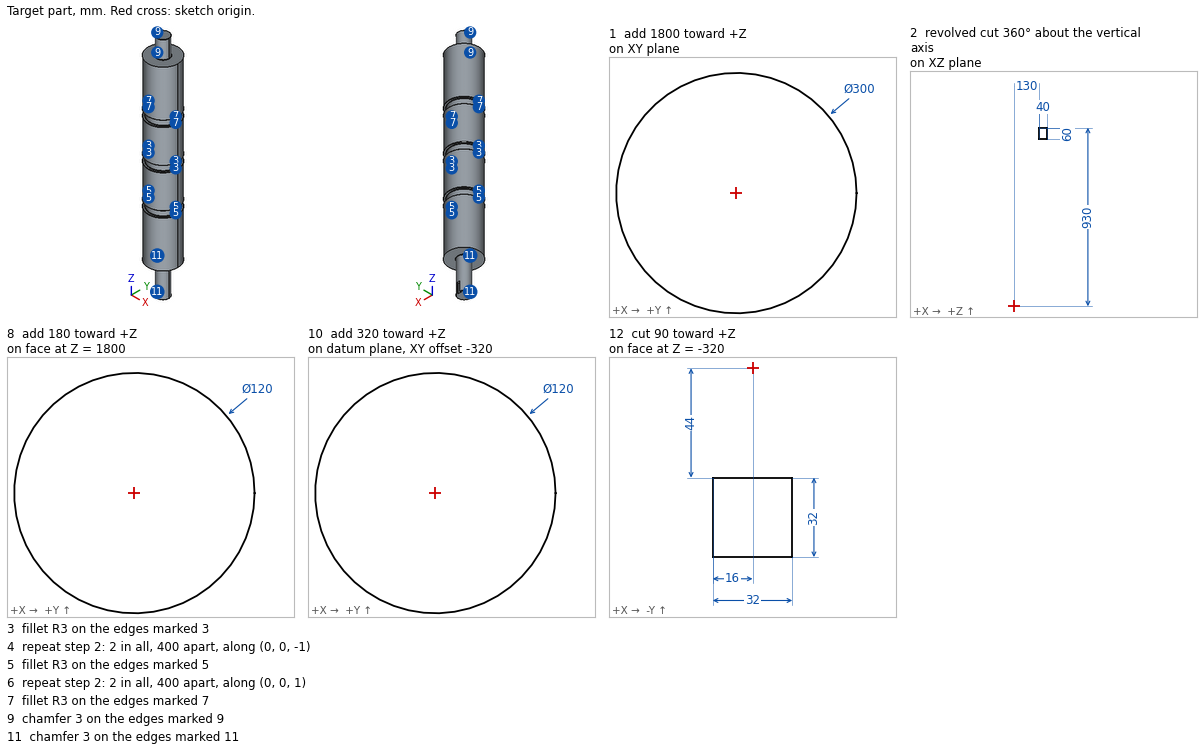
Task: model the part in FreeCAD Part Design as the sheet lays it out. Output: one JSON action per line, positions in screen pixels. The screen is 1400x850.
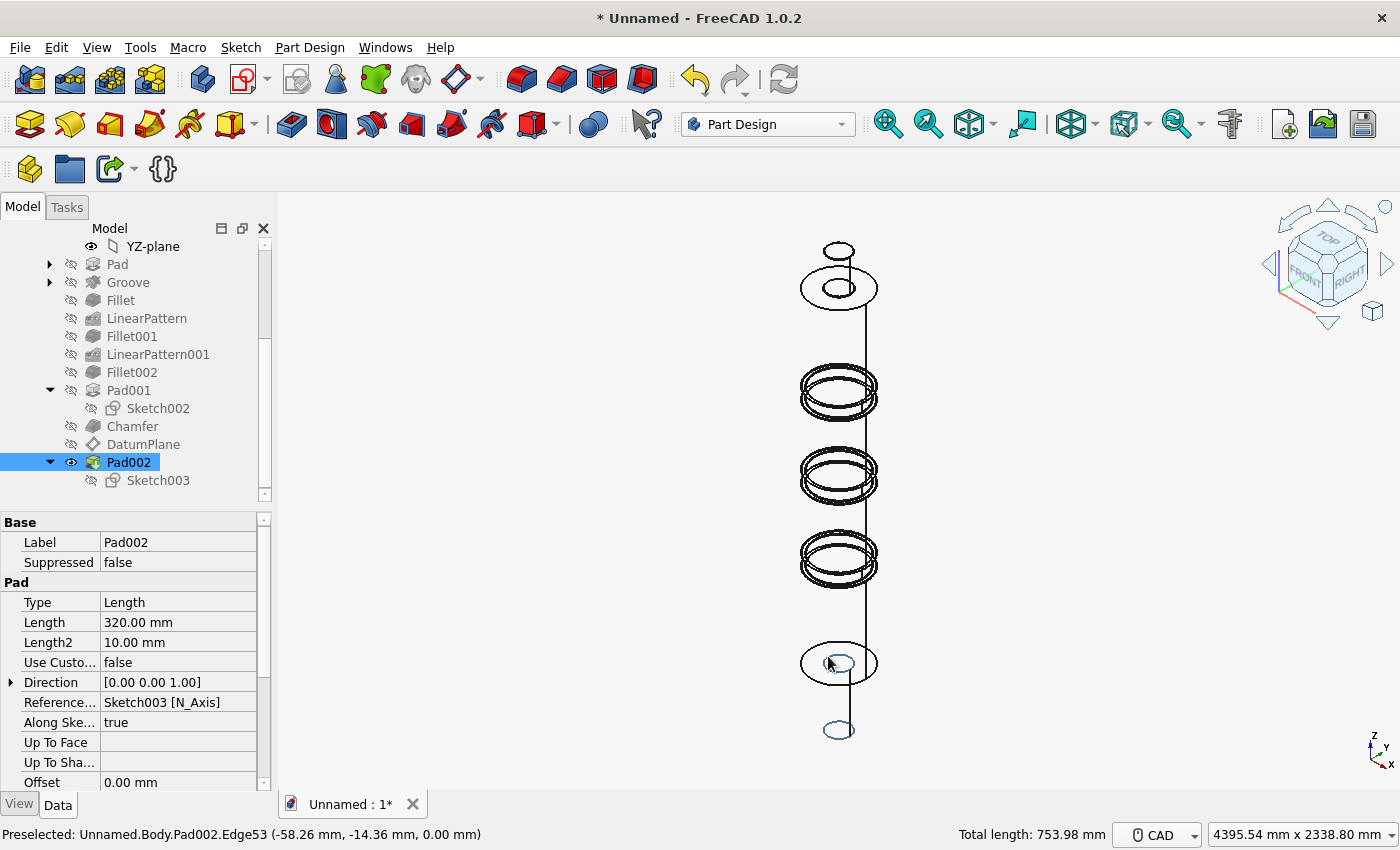
{"action": "key", "text": "v 1"}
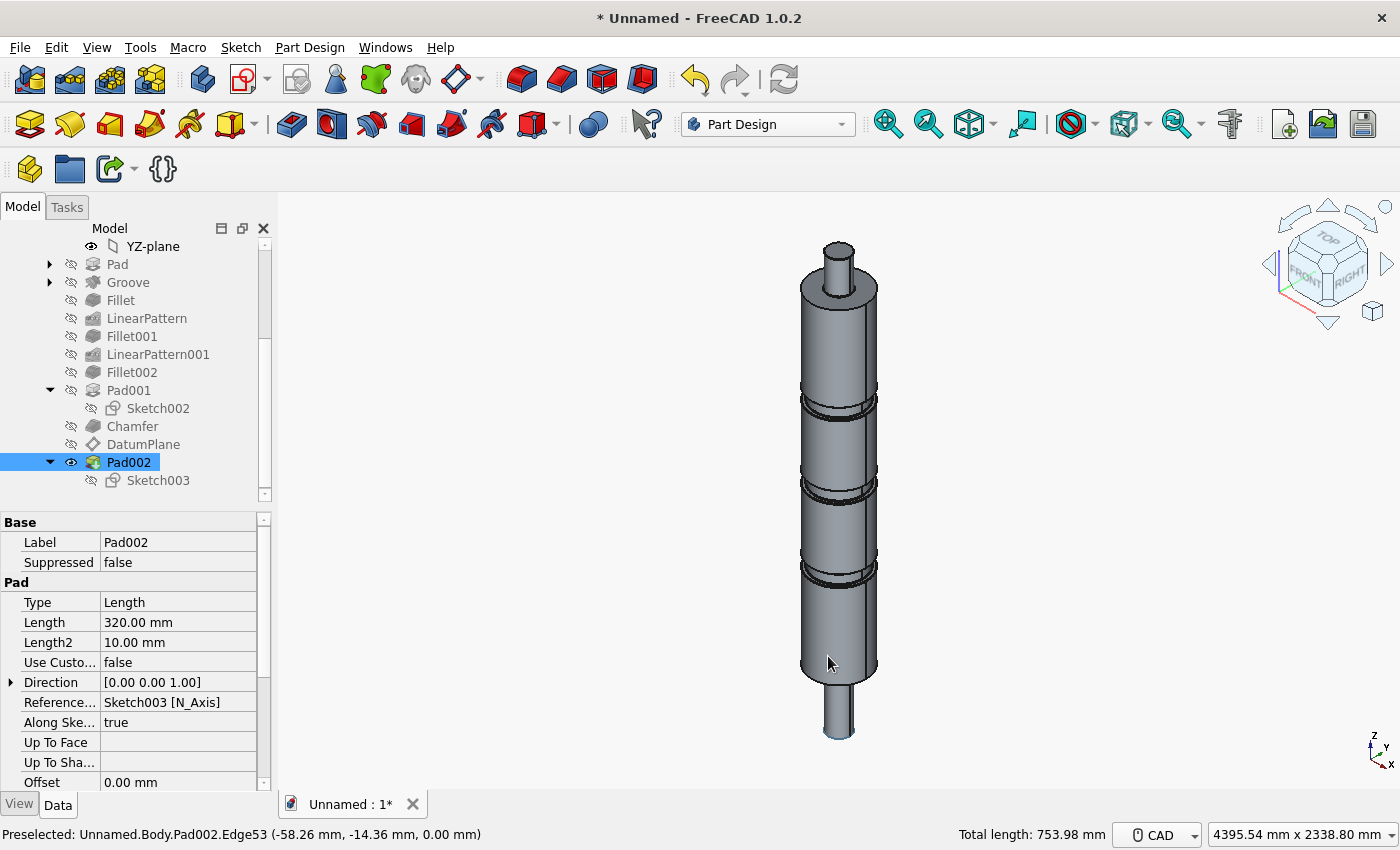
{"action": "left_click", "coordinate": [562, 80]}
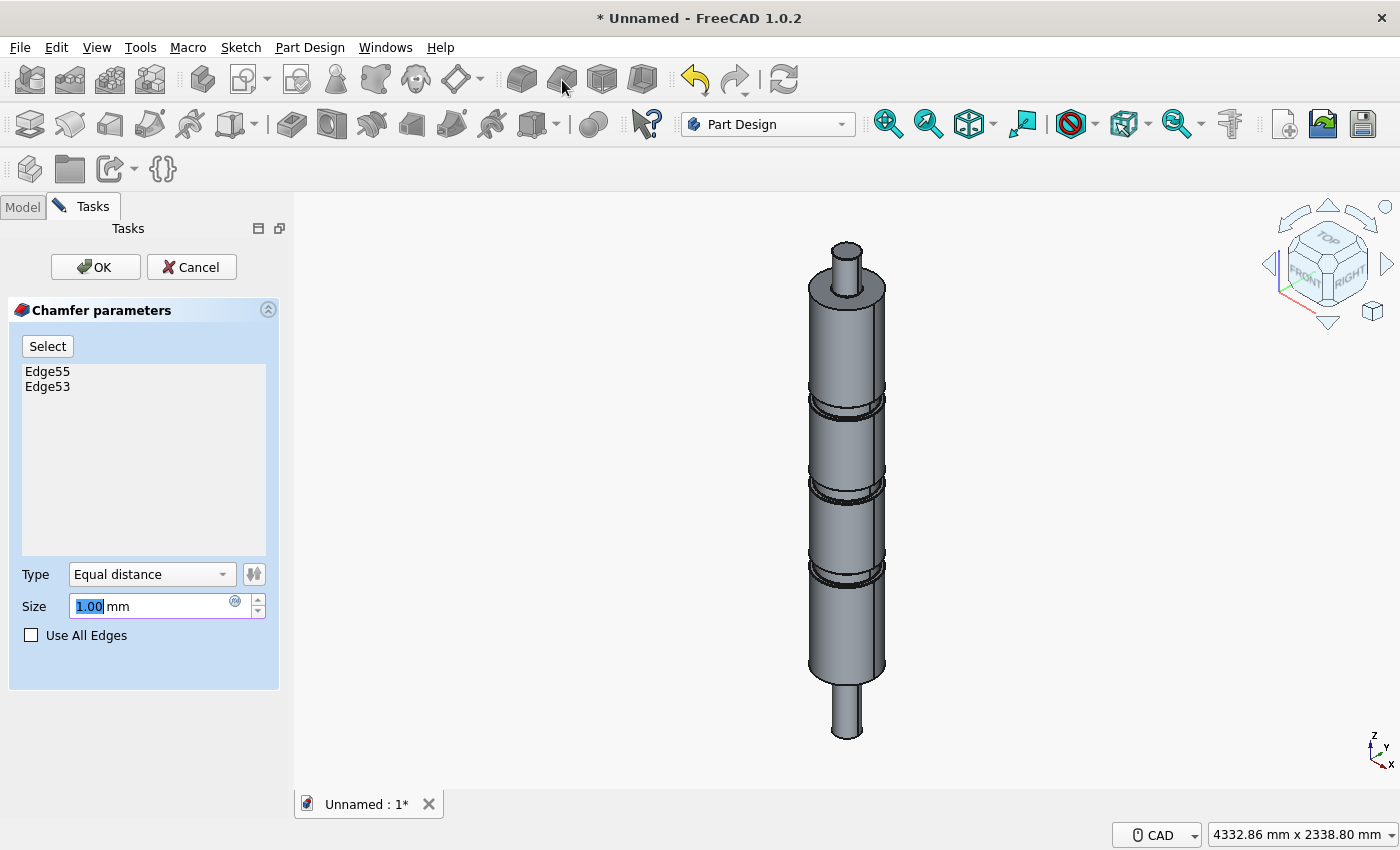
{"action": "type", "text": "3"}
{"action": "key", "text": "Tab"}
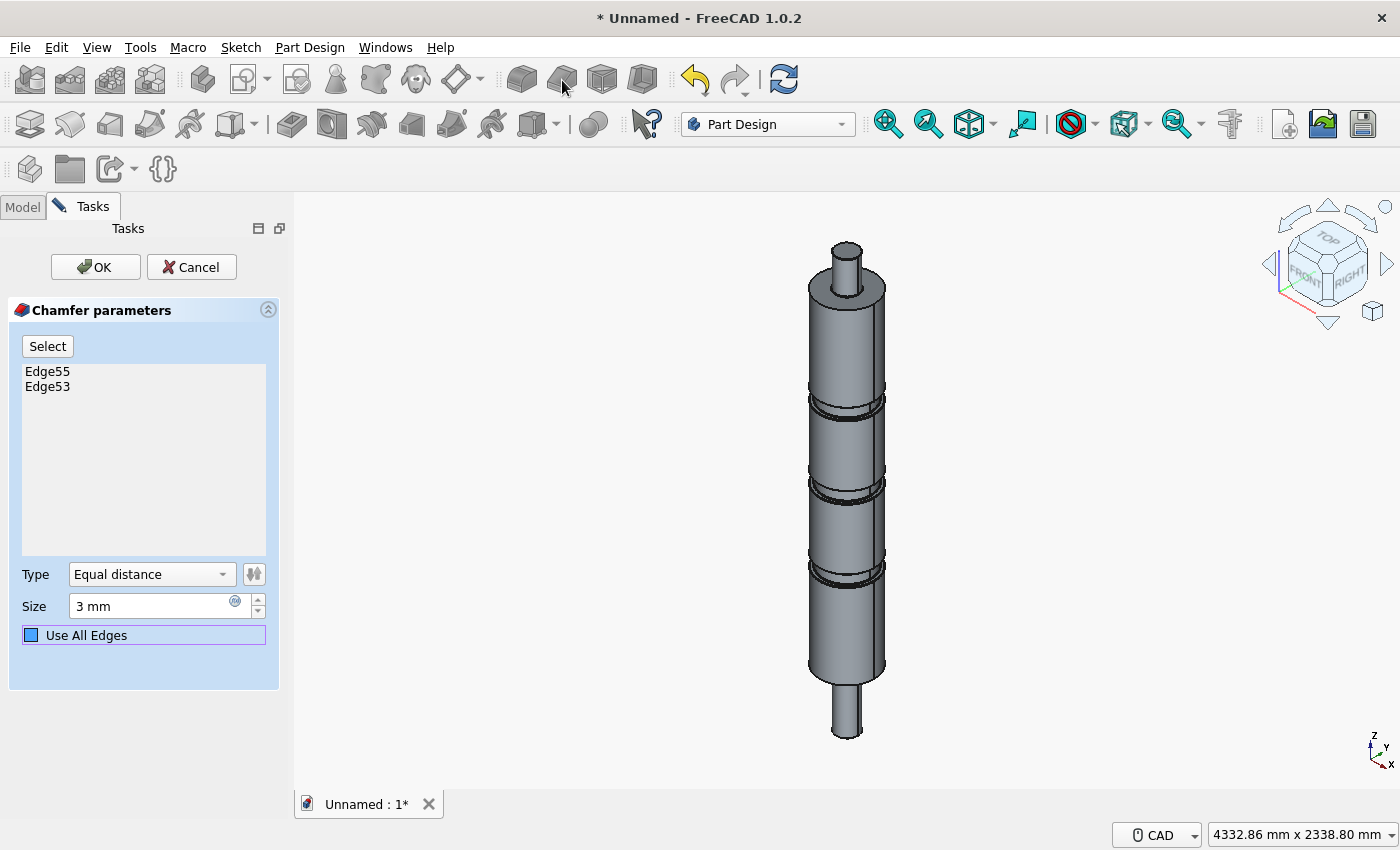
{"action": "left_click", "coordinate": [96, 267]}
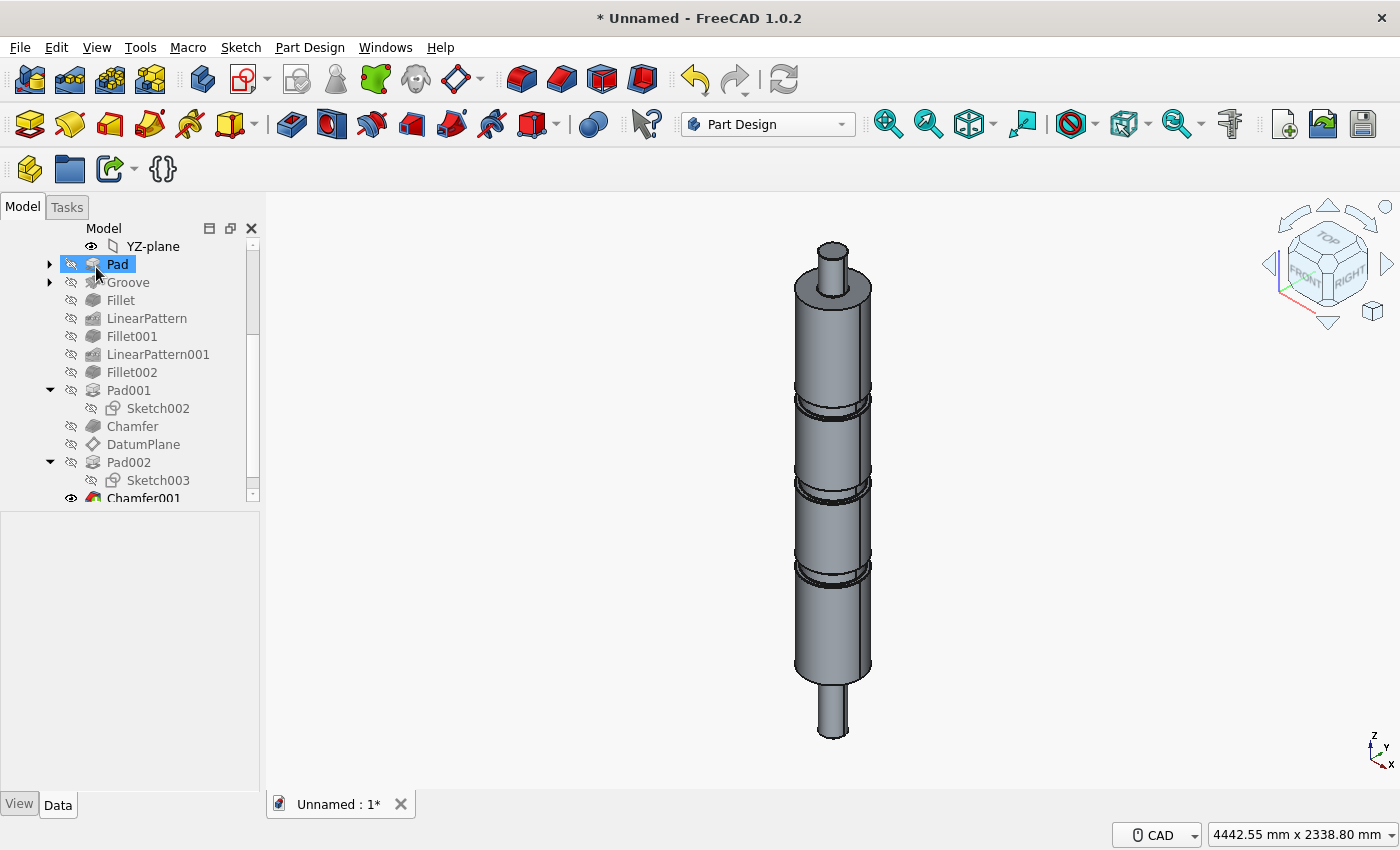
{"action": "key", "text": "5"}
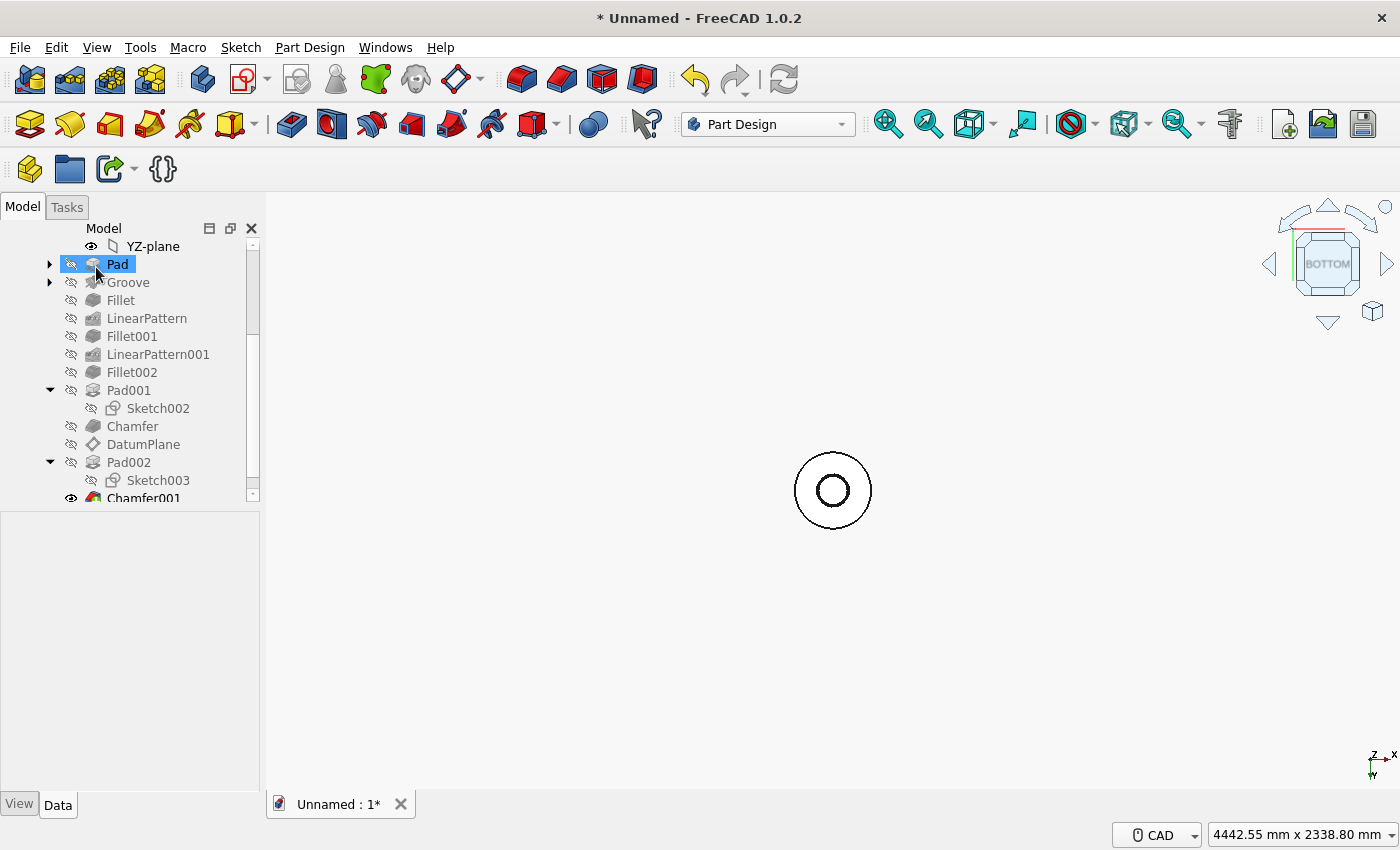
{"action": "left_click", "coordinate": [890, 124]}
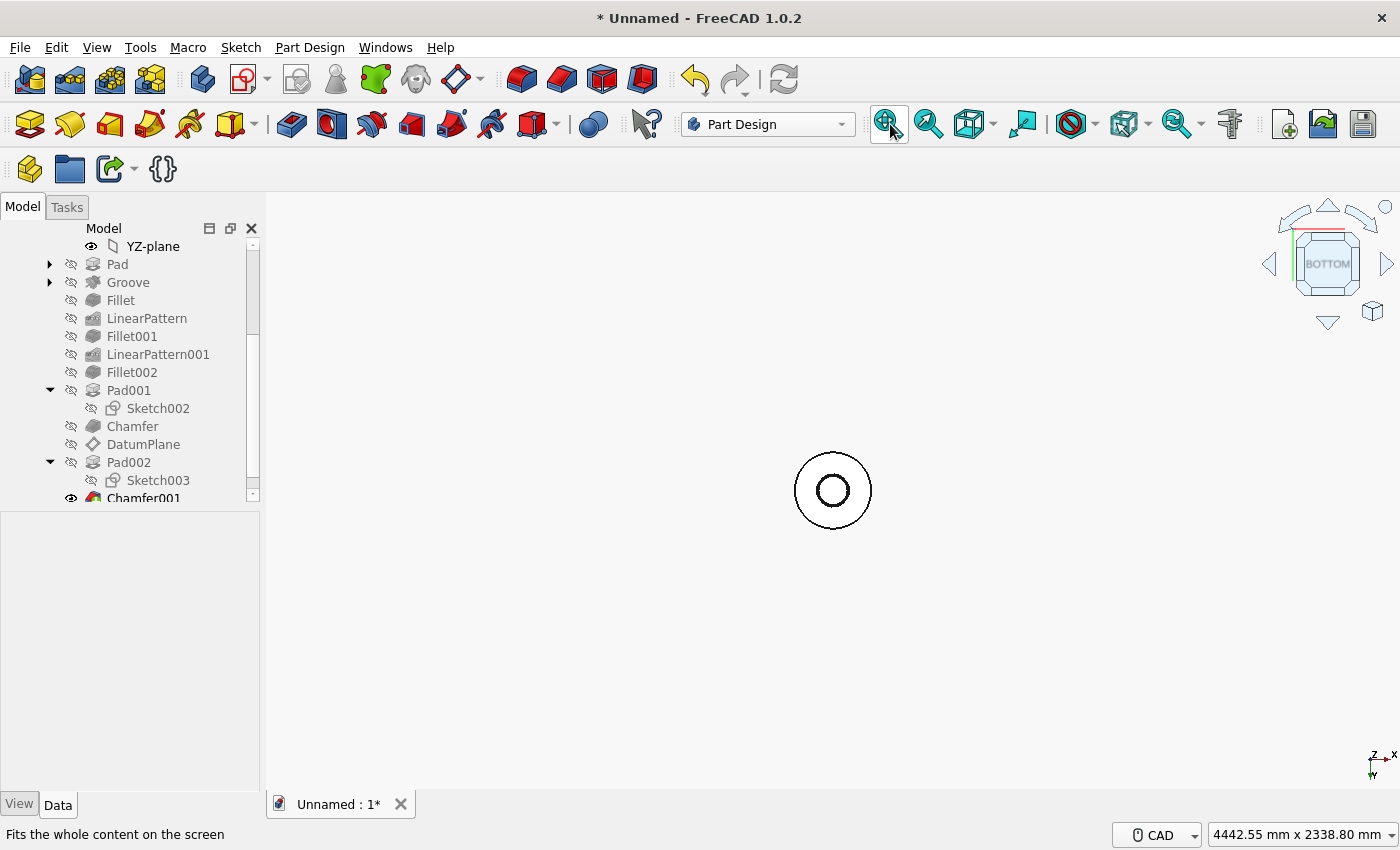
{"action": "left_click", "coordinate": [833, 489]}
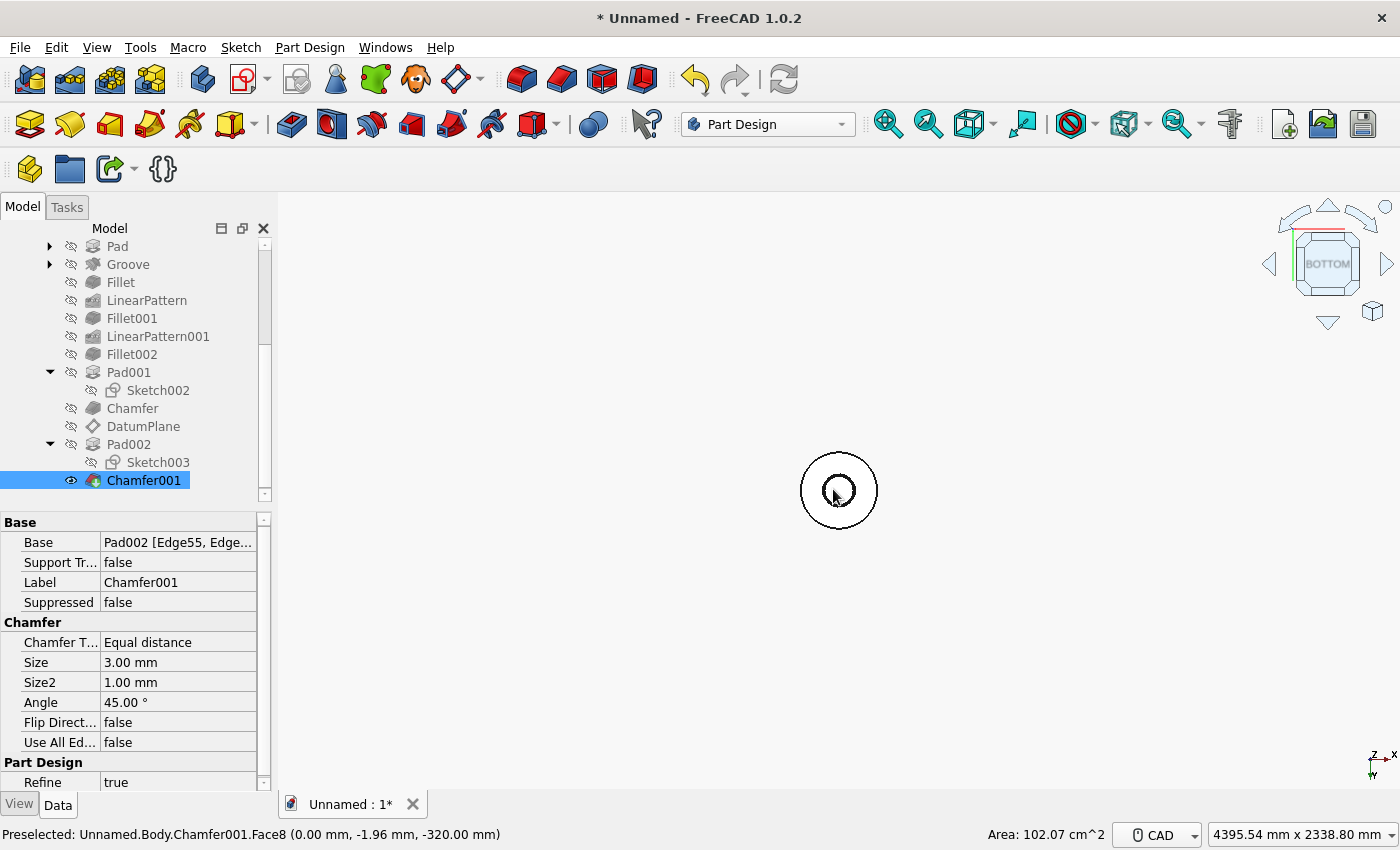
{"action": "left_click", "coordinate": [244, 80]}